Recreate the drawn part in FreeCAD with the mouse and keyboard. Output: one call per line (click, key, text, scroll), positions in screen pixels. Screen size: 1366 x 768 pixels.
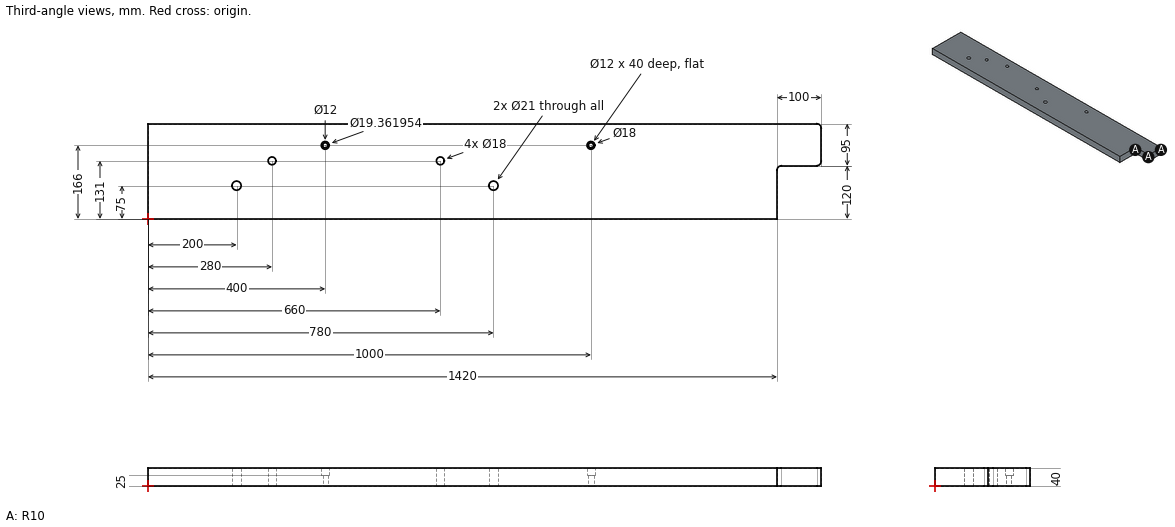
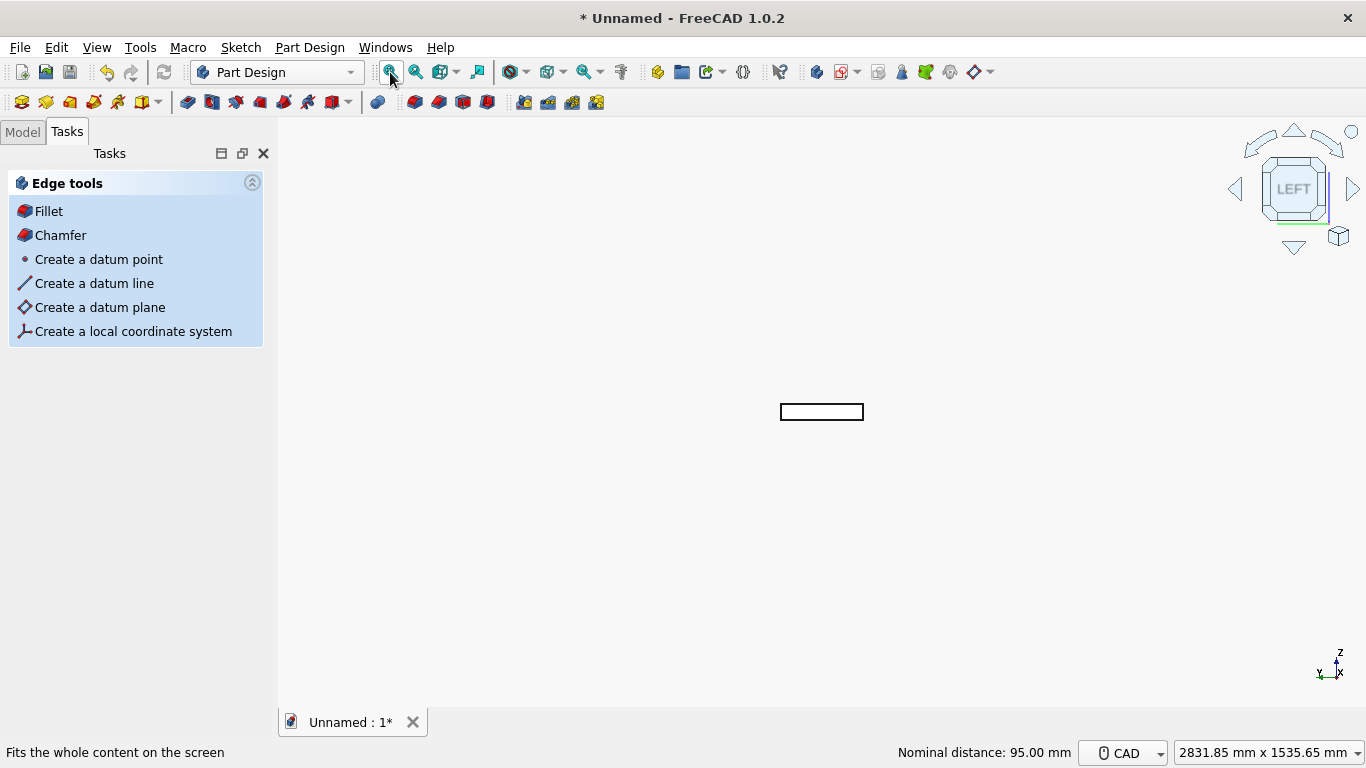
scroll(817, 411, up, 5)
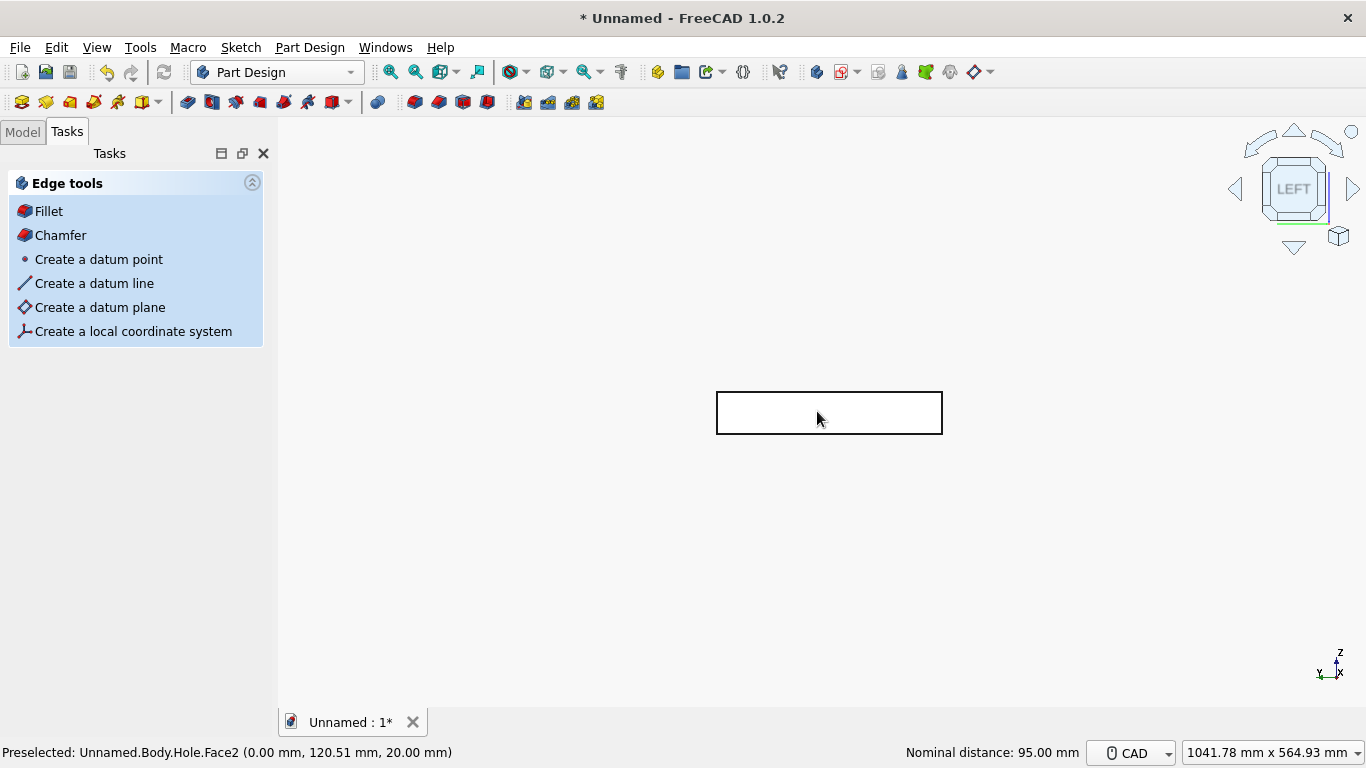
key(v)
key(f)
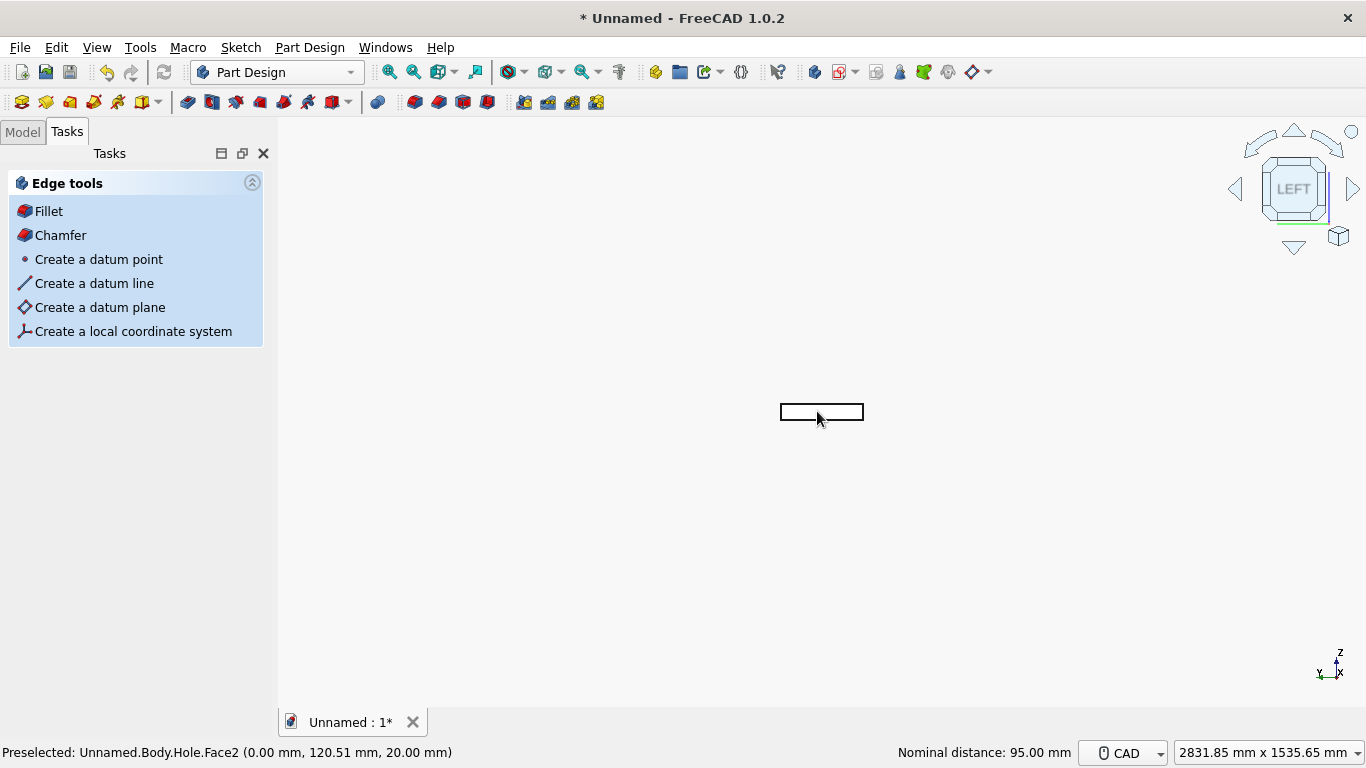
key(v)
key(3)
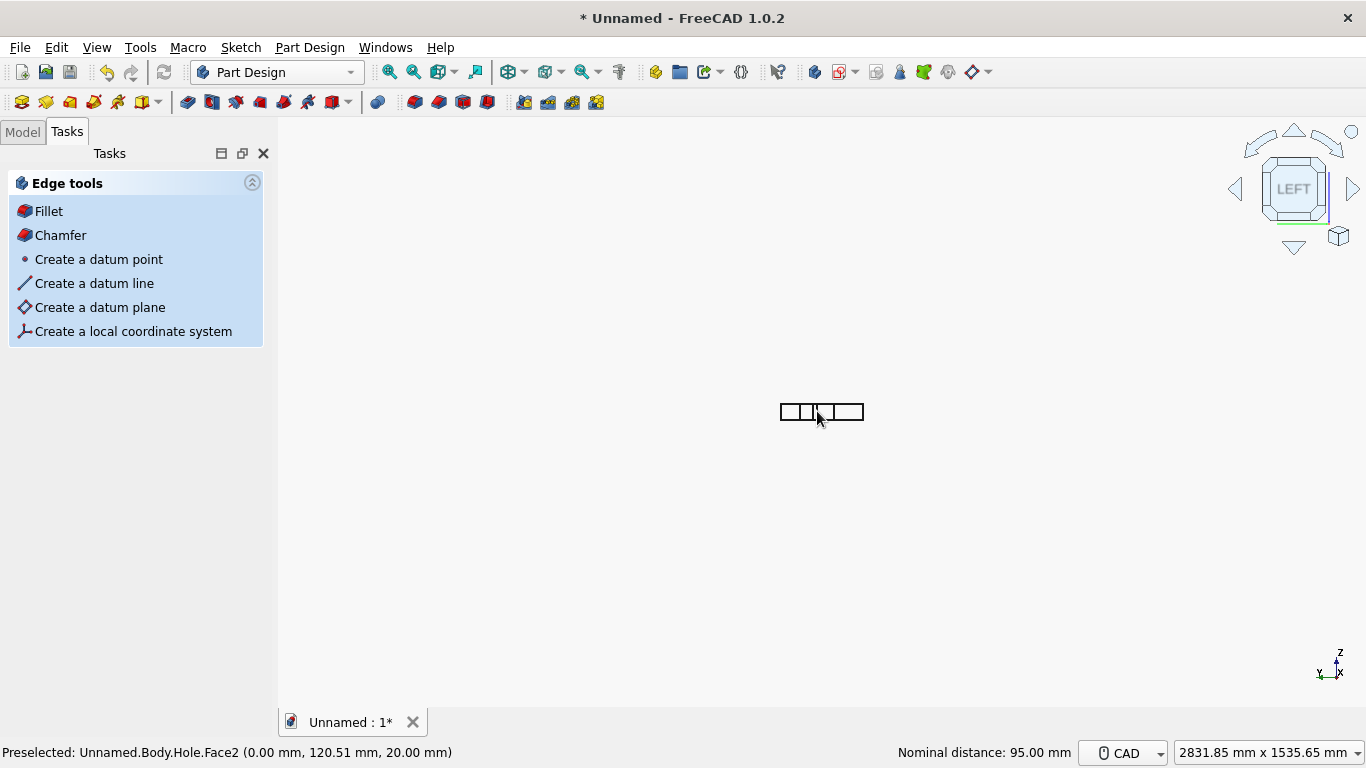
key(0)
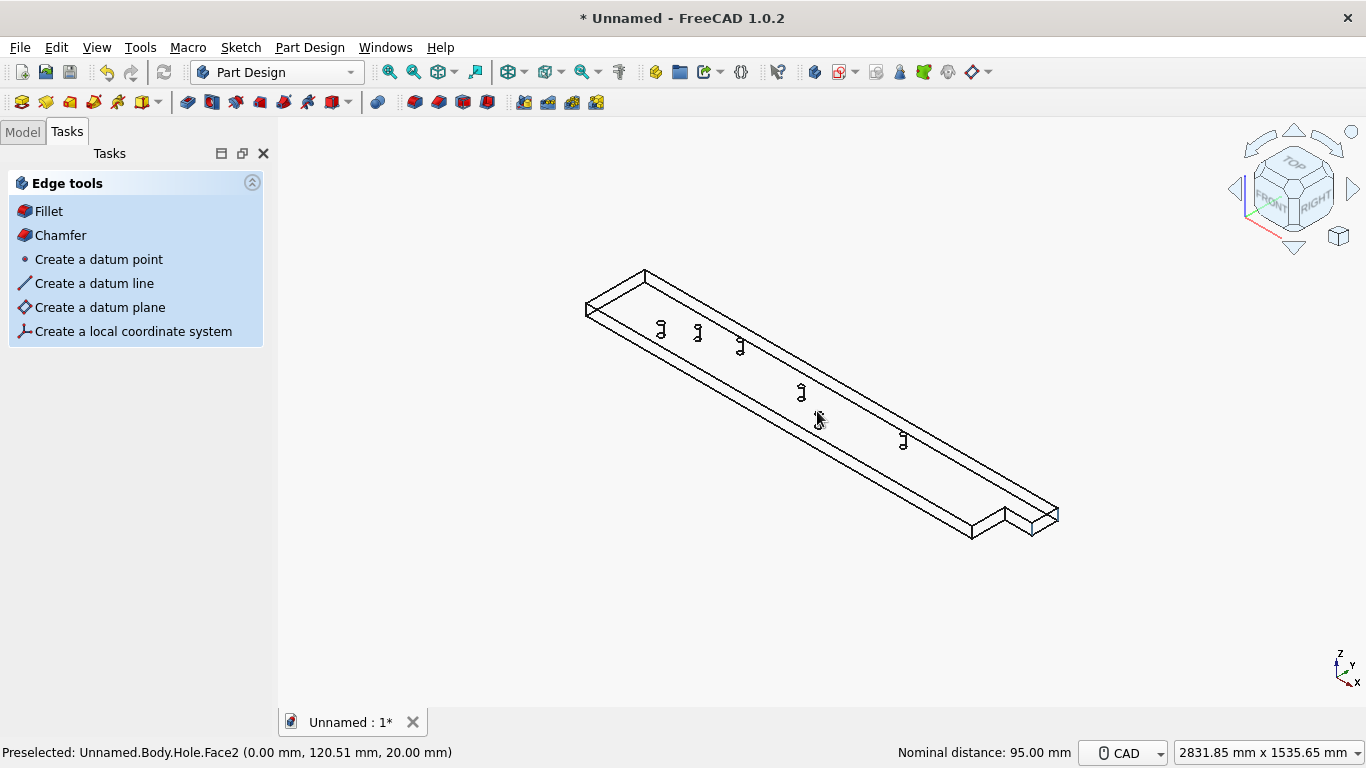
click(1005, 514, ctrl)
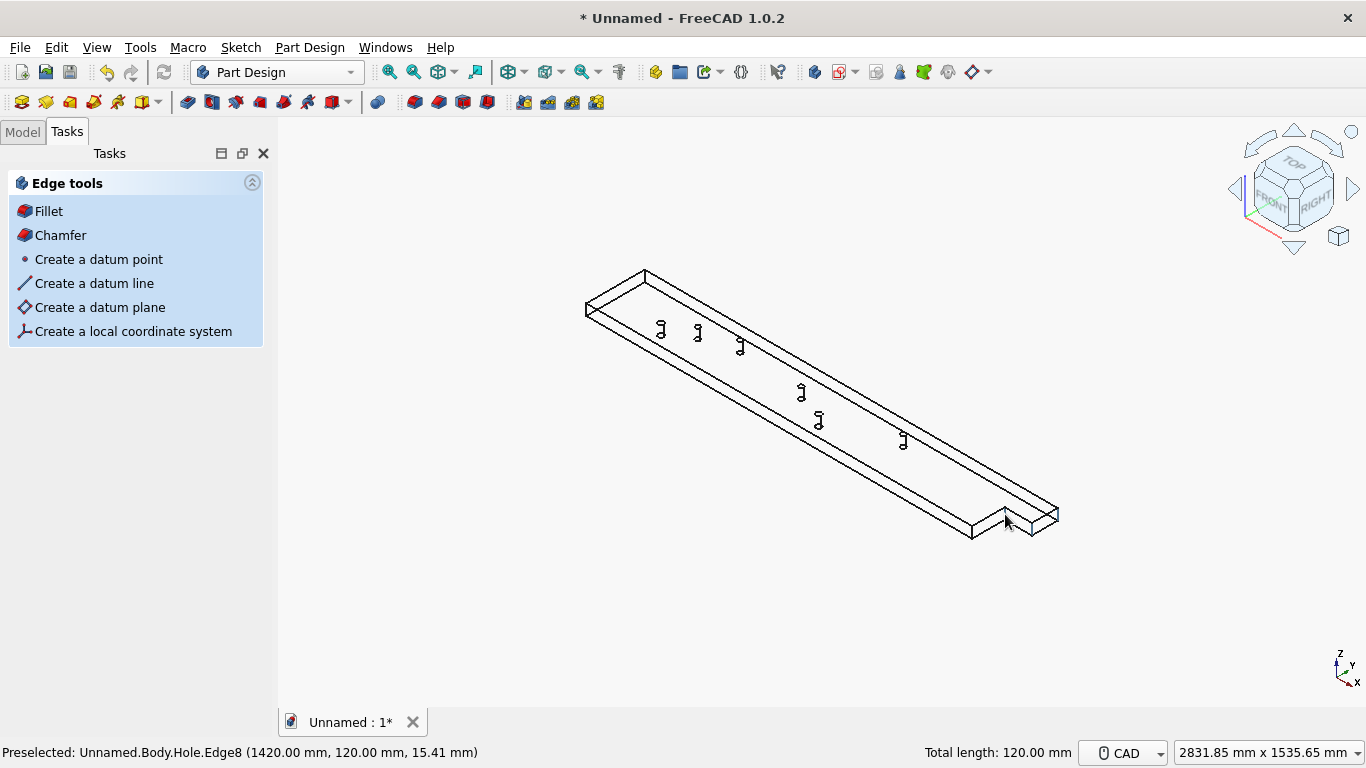
key(v)
key(1)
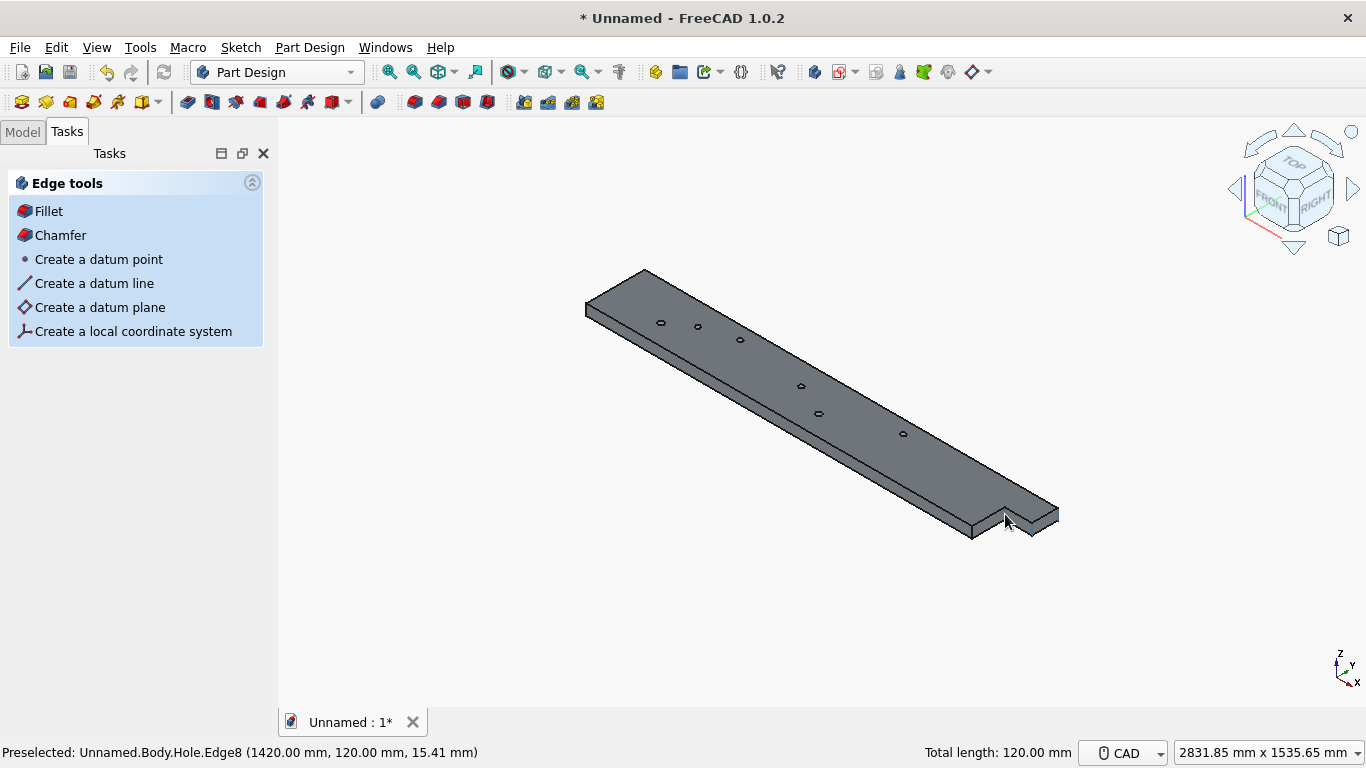
click(416, 102)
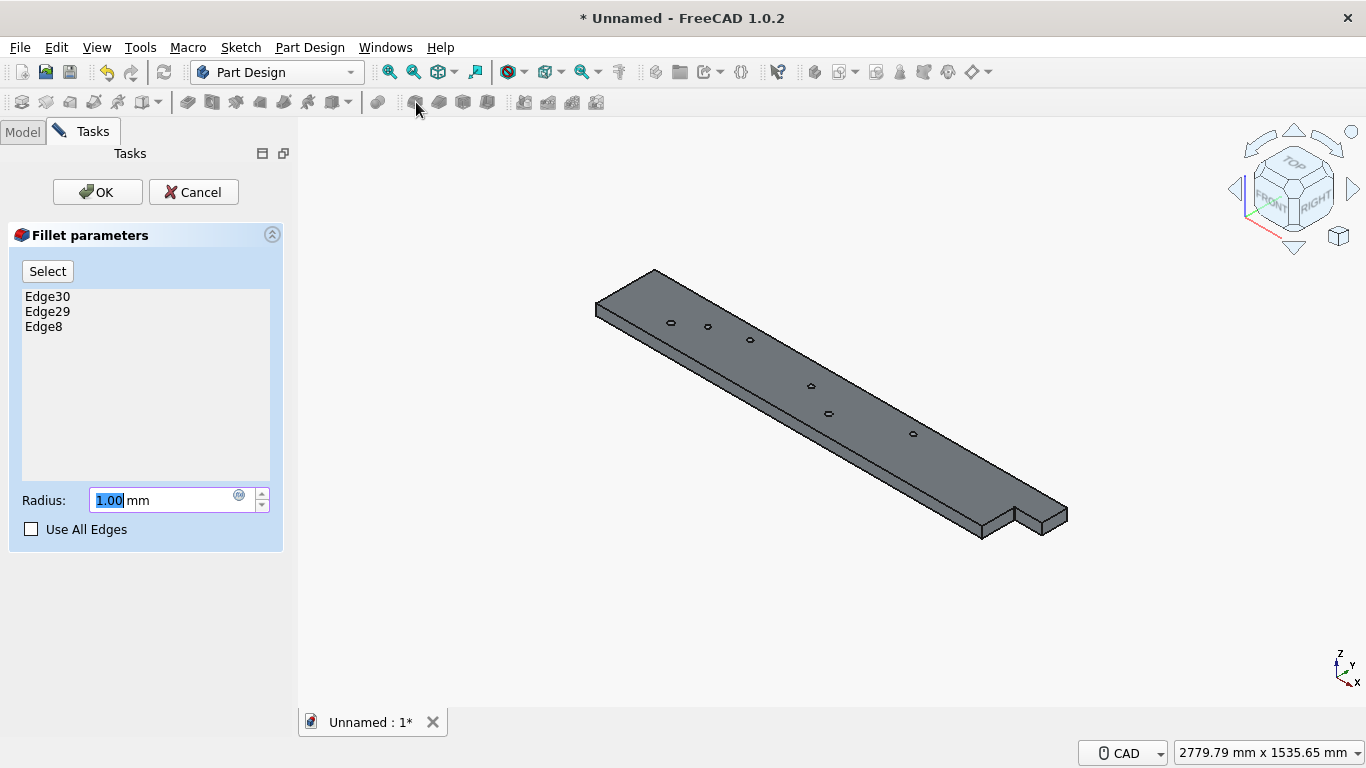
text(10)
key(Tab)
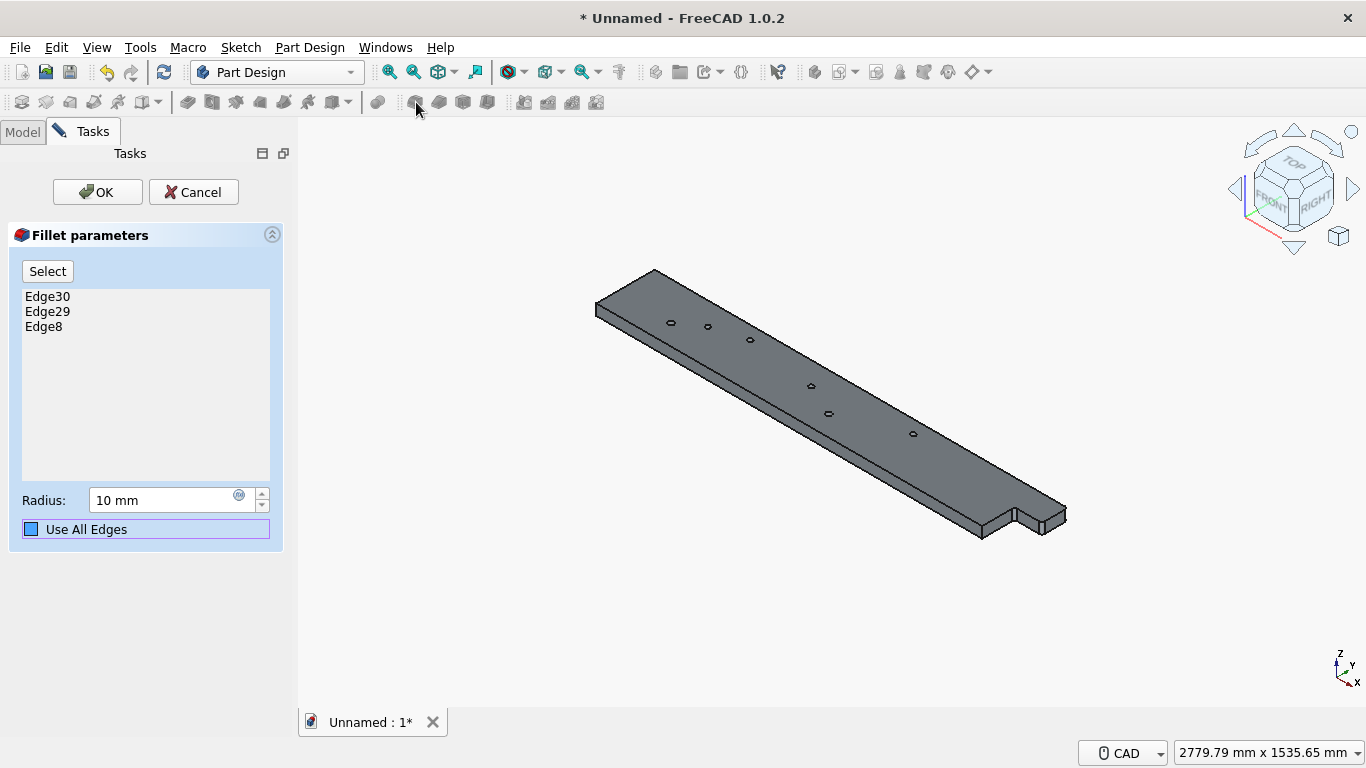
click(98, 192)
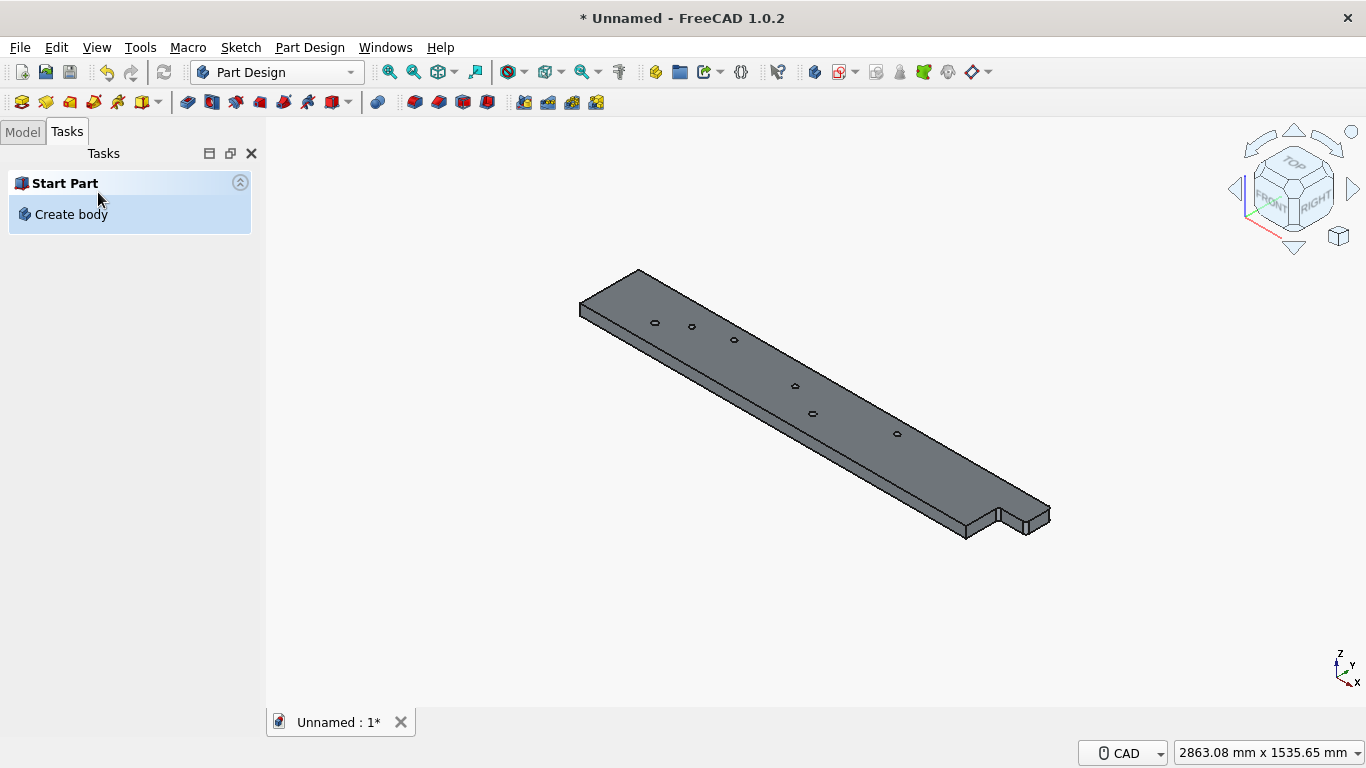
click(840, 72)